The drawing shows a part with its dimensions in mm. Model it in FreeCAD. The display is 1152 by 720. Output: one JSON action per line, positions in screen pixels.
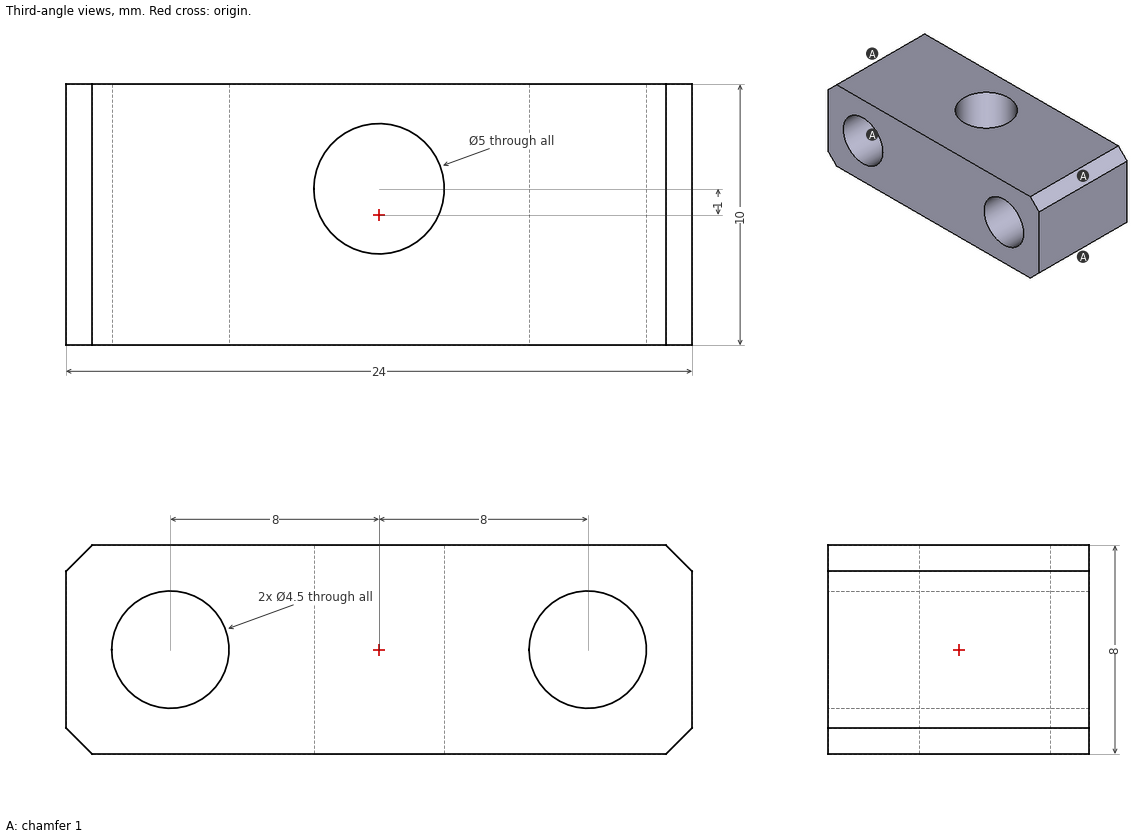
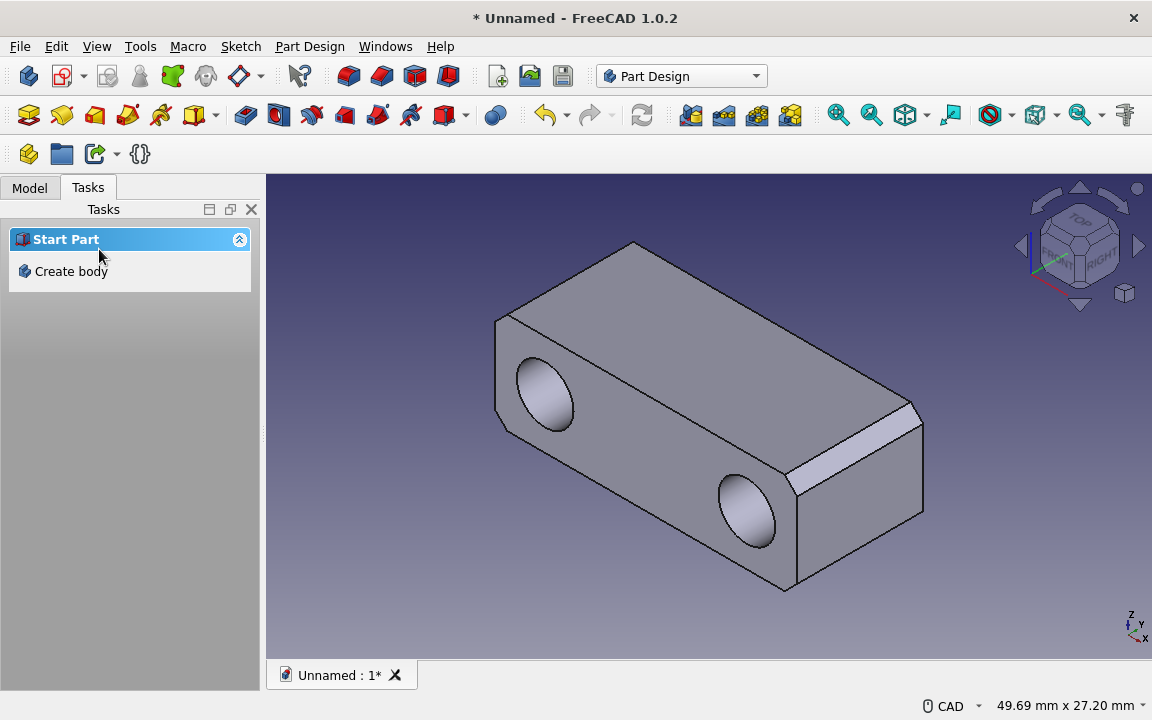
{"action": "left_click", "coordinate": [749, 380]}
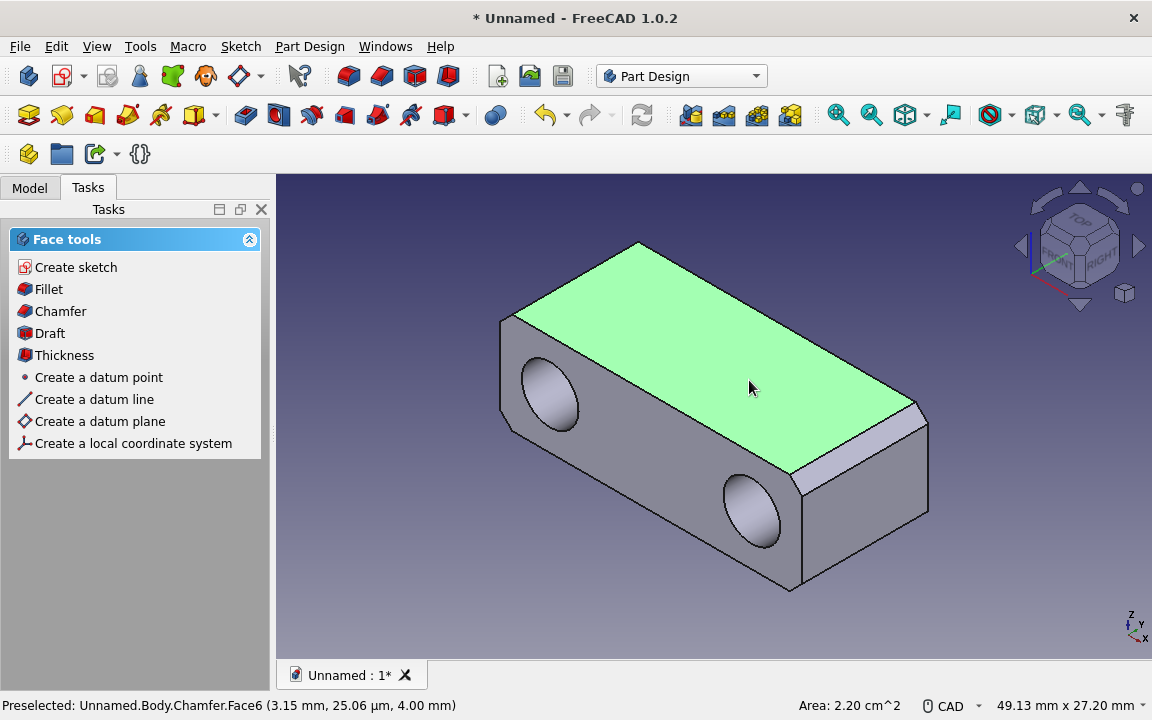
{"action": "left_click", "coordinate": [62, 76]}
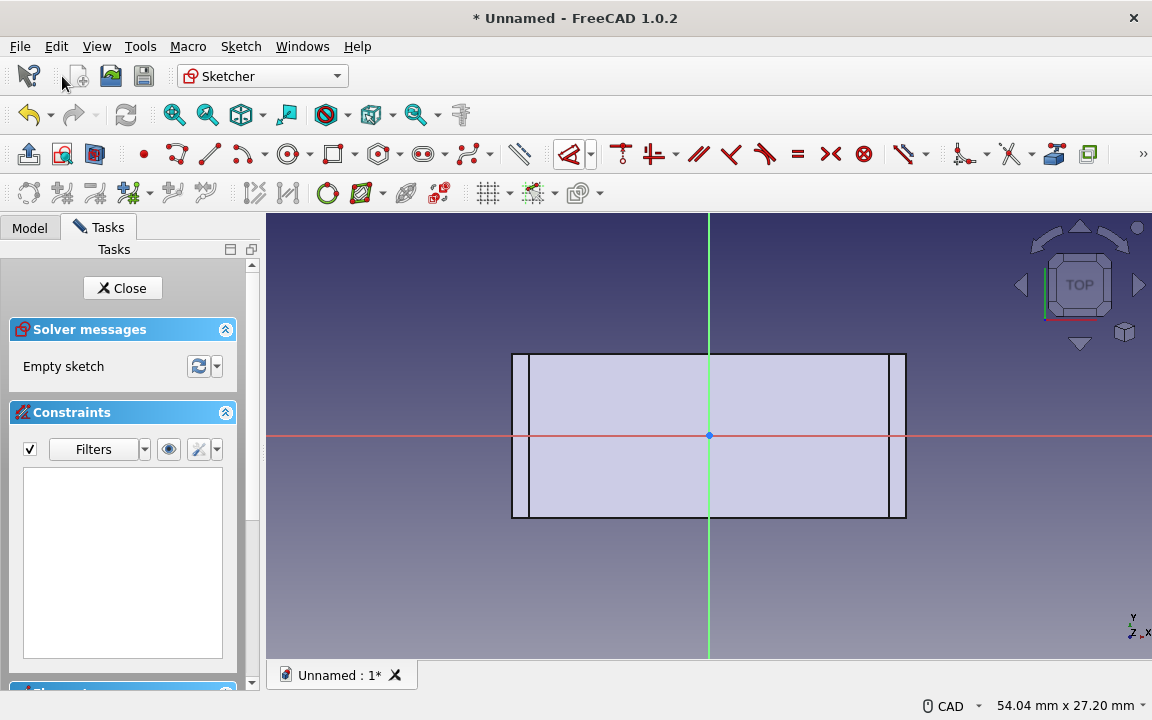
{"action": "scroll", "coordinate": [739, 413], "scroll_direction": "up", "scroll_amount": 6}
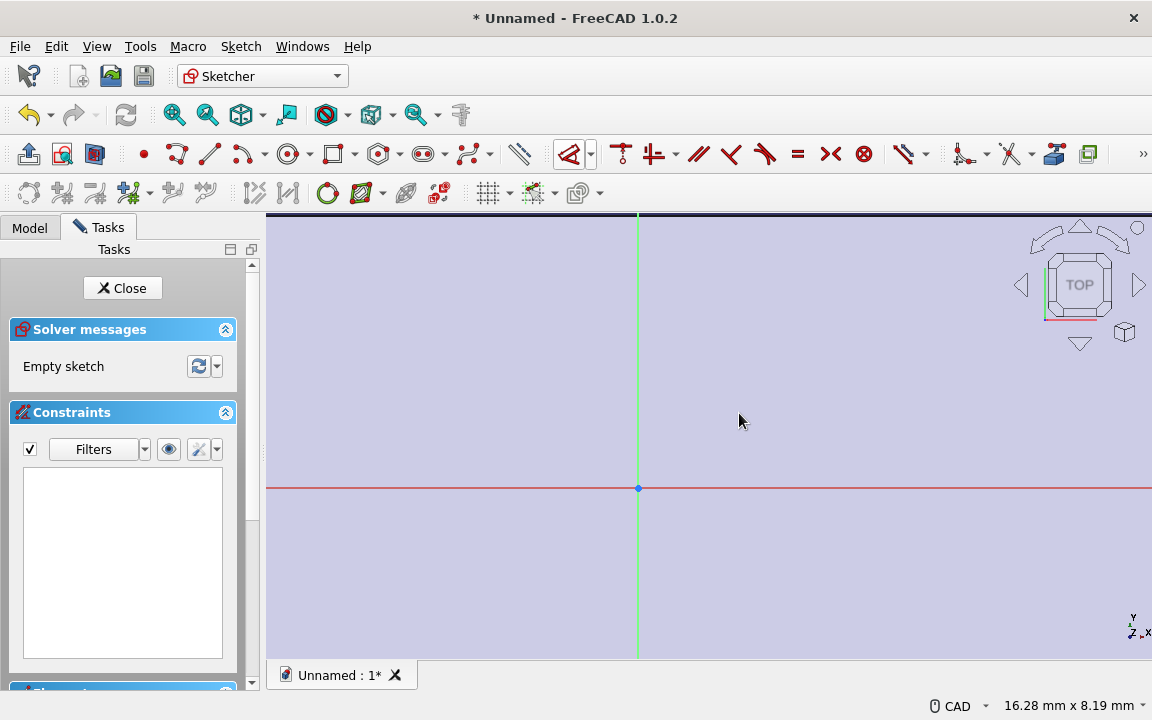
{"action": "left_click", "coordinate": [288, 154]}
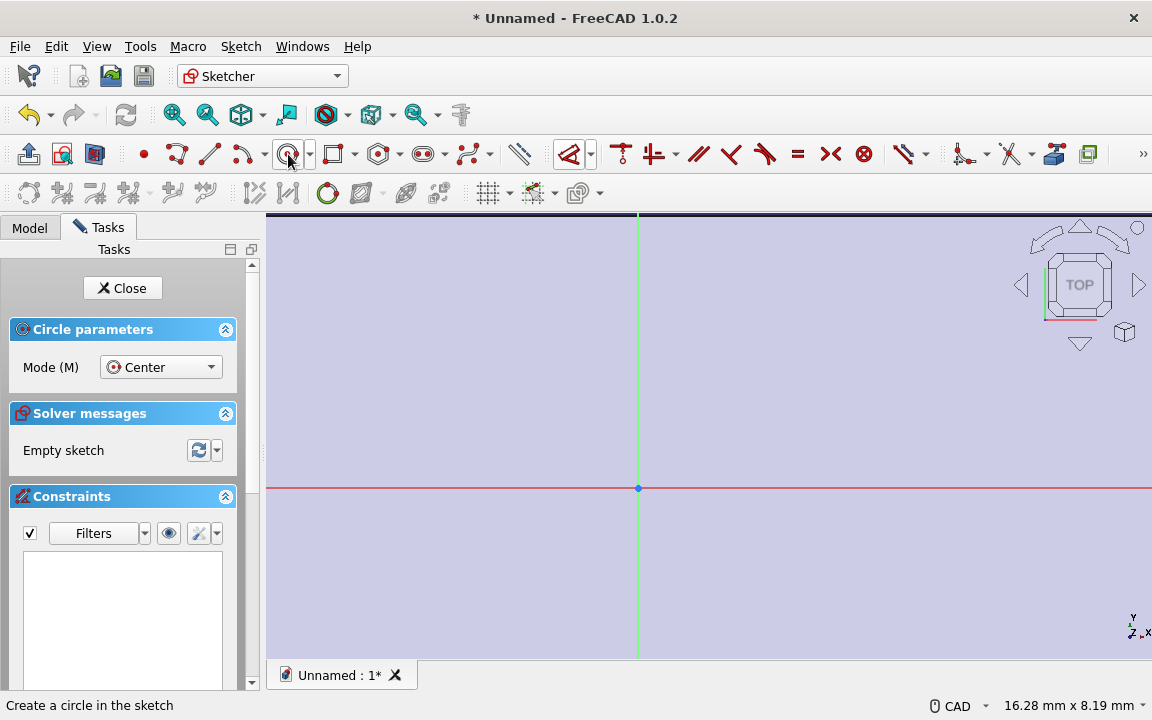
{"action": "left_click", "coordinate": [638, 434]}
{"action": "left_click", "coordinate": [734, 338]}
{"action": "key", "text": "Escape"}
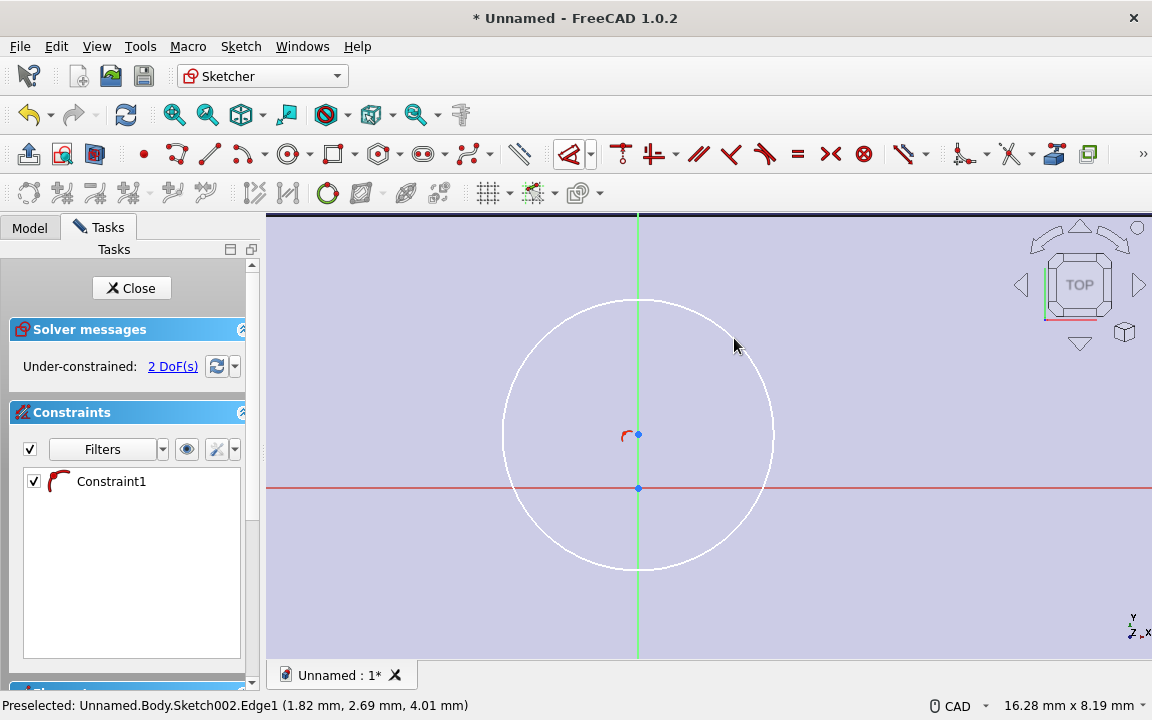
{"action": "left_click", "coordinate": [734, 339]}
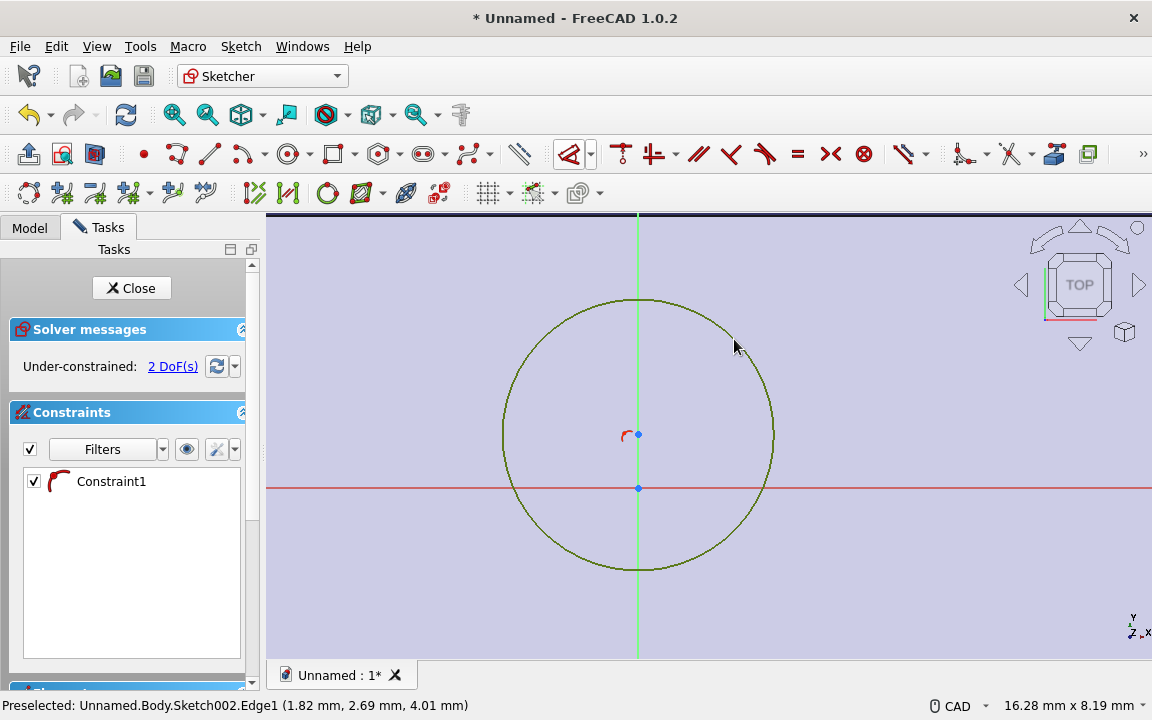
{"action": "left_click", "coordinate": [590, 154]}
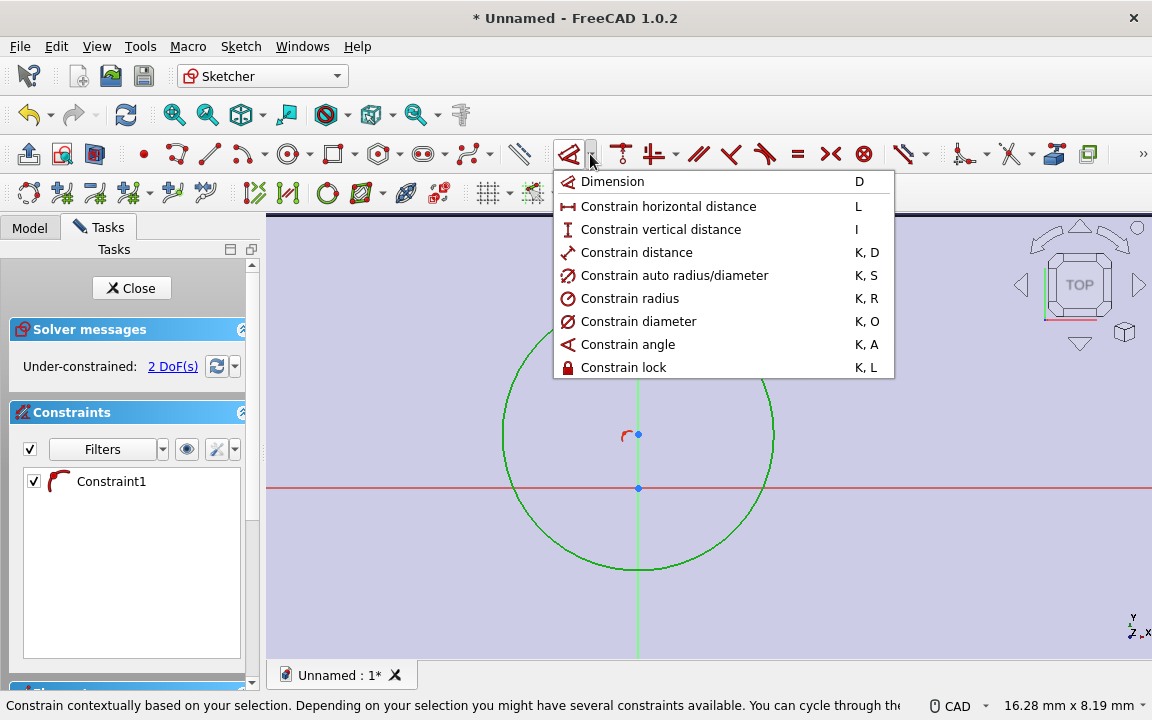
{"action": "left_click", "coordinate": [724, 322]}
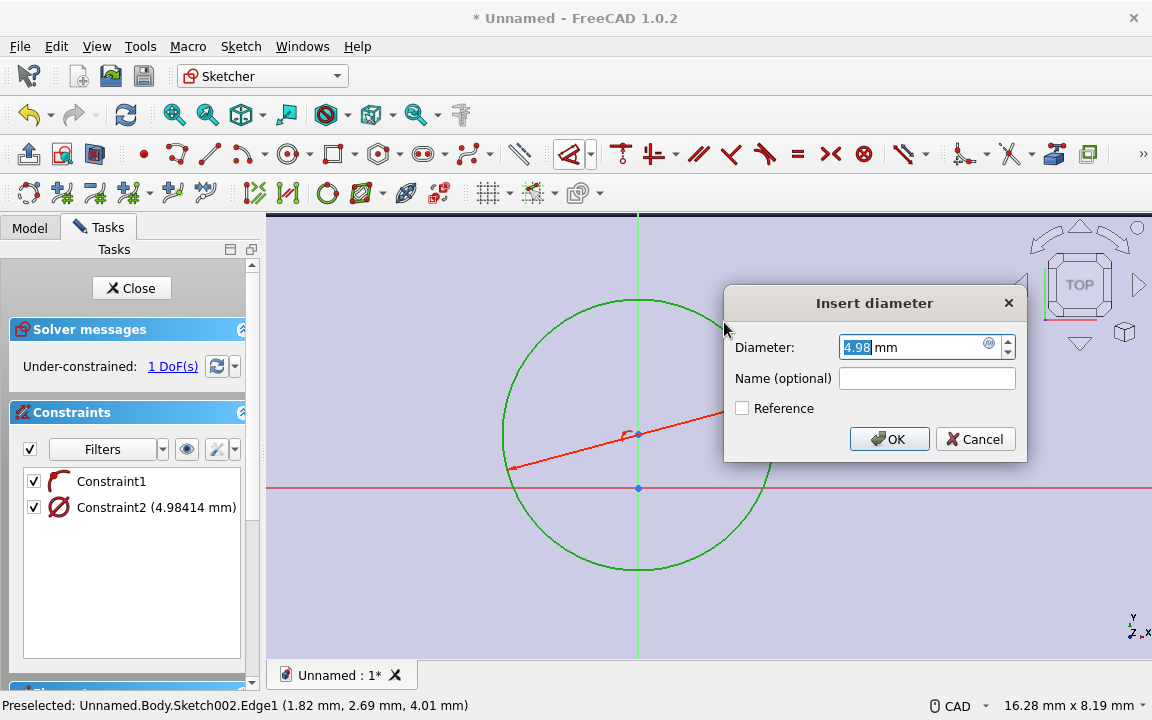
{"action": "type", "text": "5"}
{"action": "key", "text": "Return"}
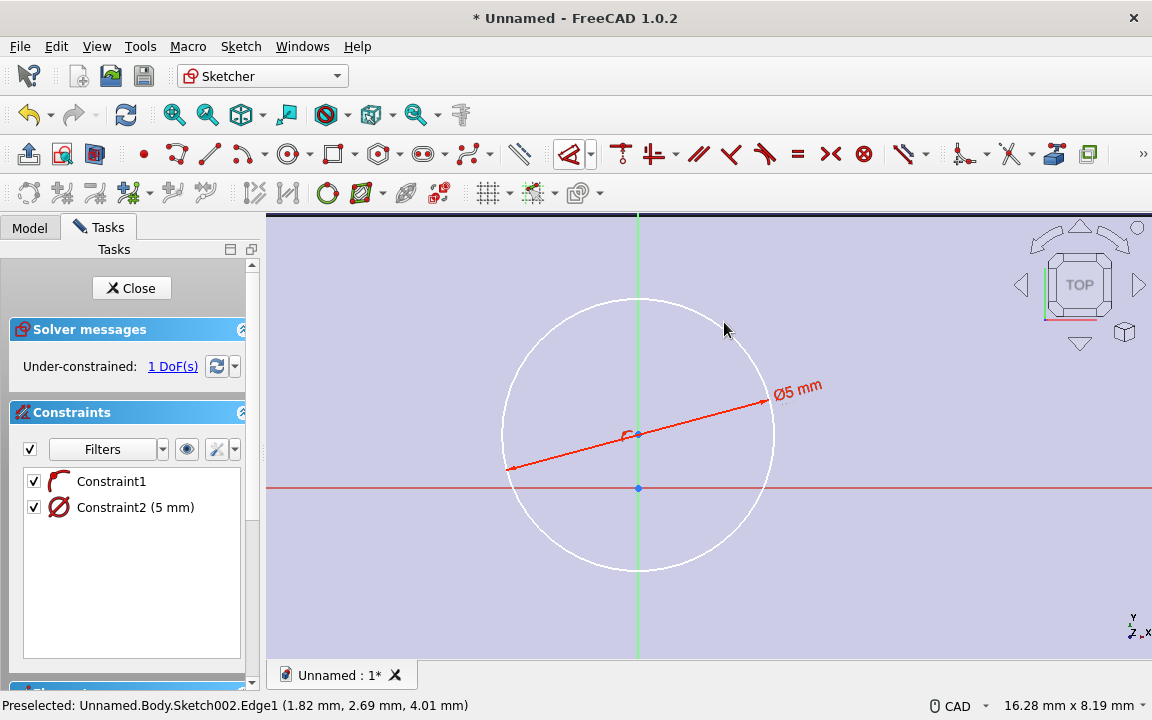
{"action": "left_click", "coordinate": [638, 435]}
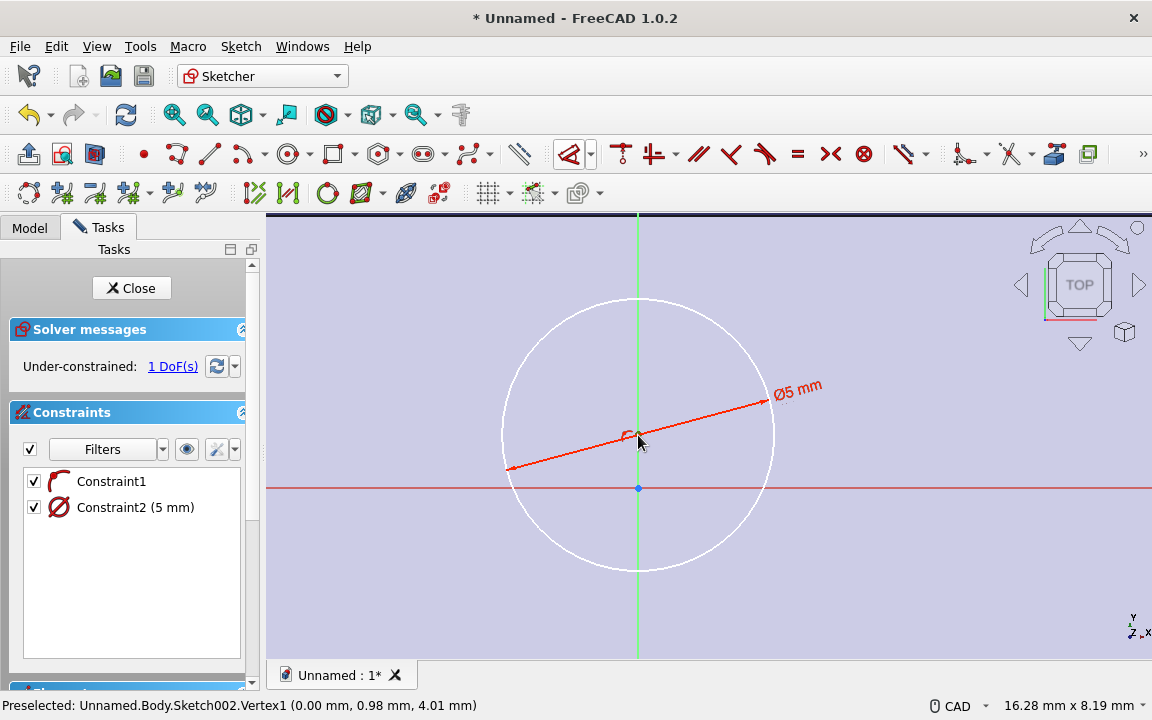
{"action": "left_click", "coordinate": [590, 154]}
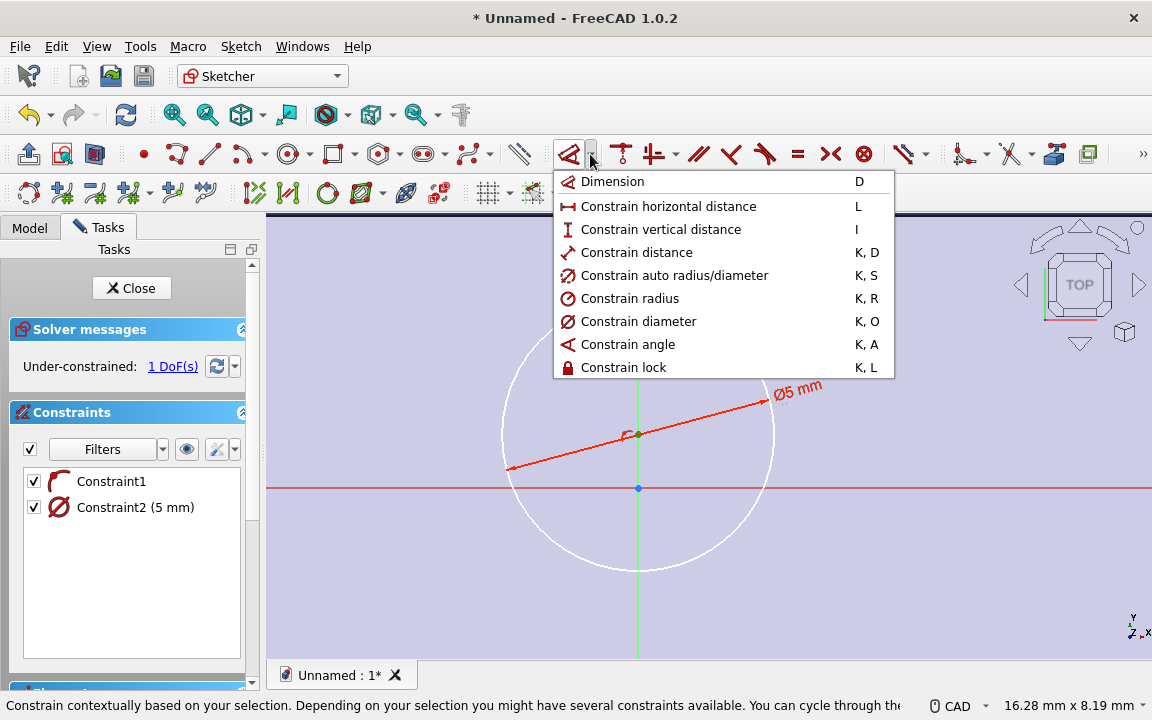
{"action": "left_click", "coordinate": [724, 230]}